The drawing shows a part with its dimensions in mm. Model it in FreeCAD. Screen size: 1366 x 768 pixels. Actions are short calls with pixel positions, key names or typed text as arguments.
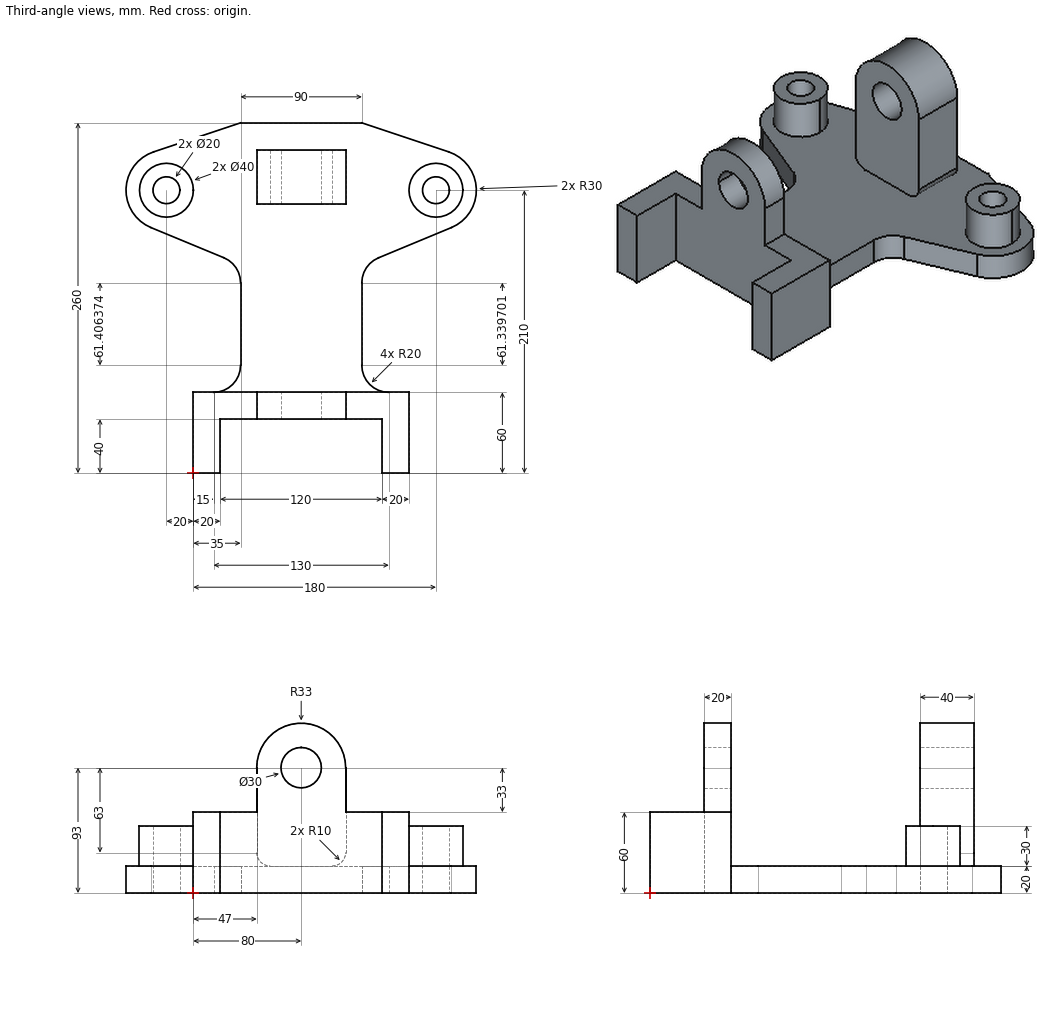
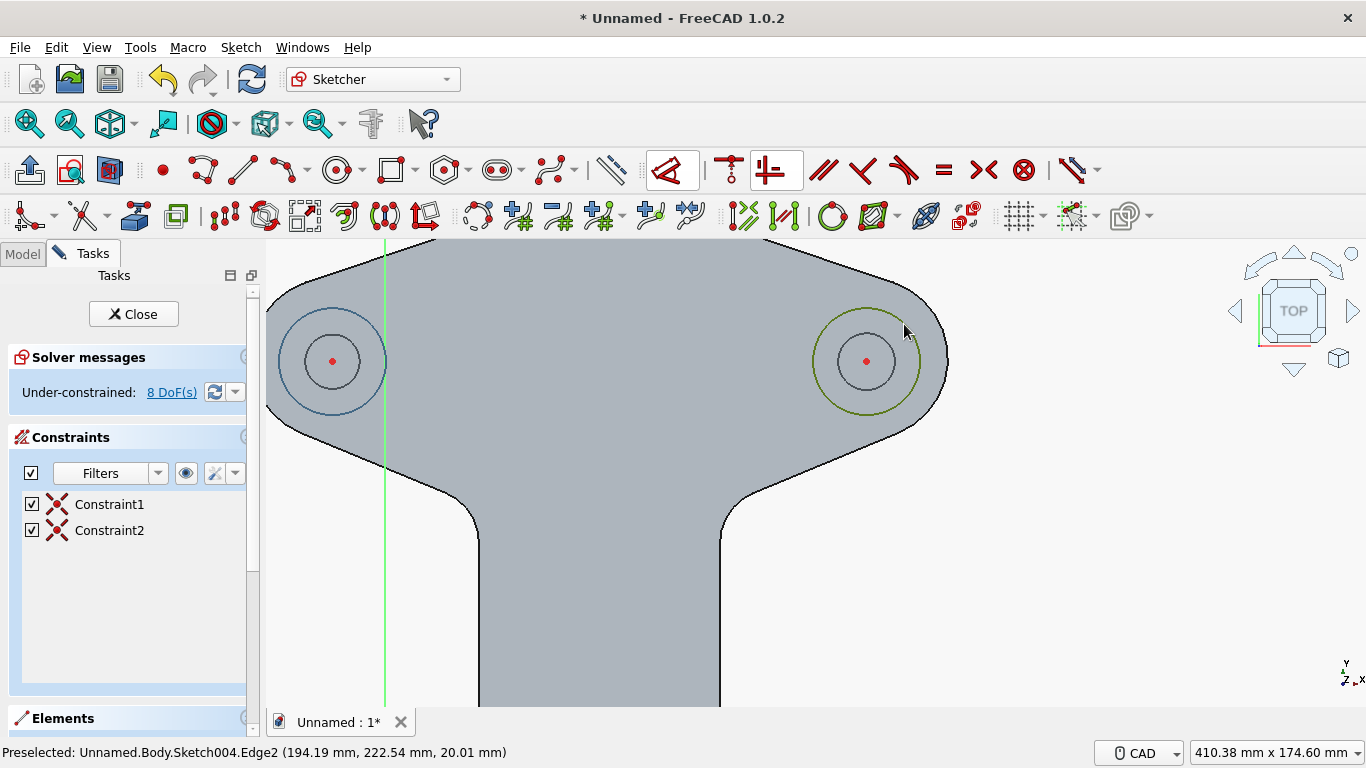
key(e)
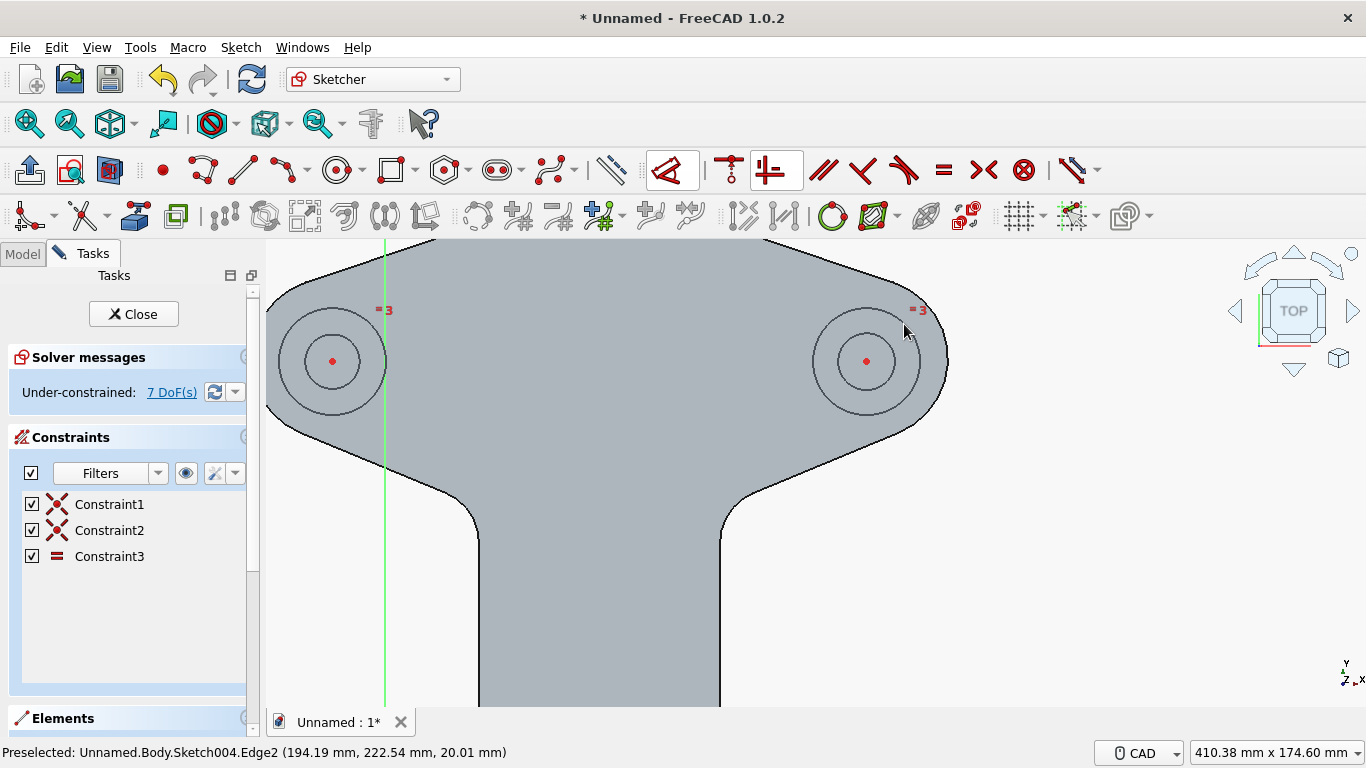
click(352, 342)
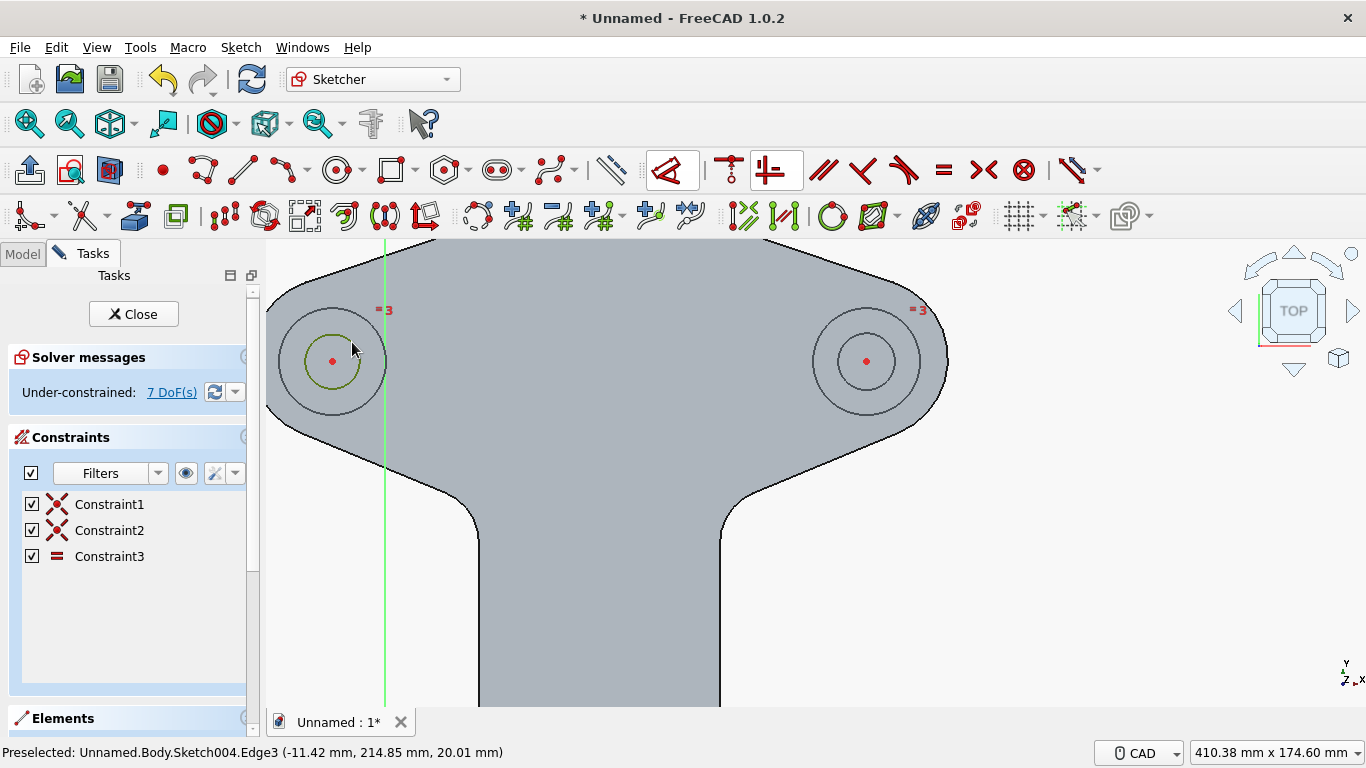
click(887, 342)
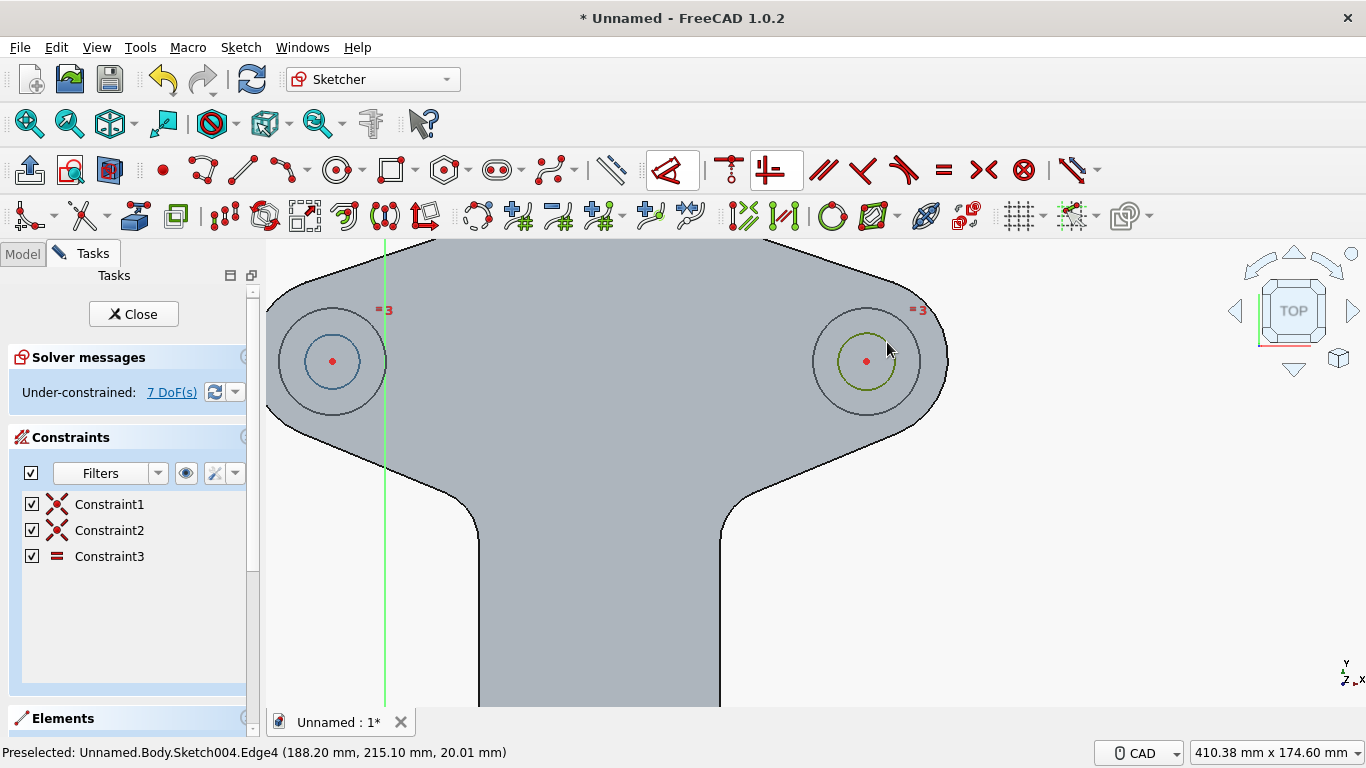
click(944, 170)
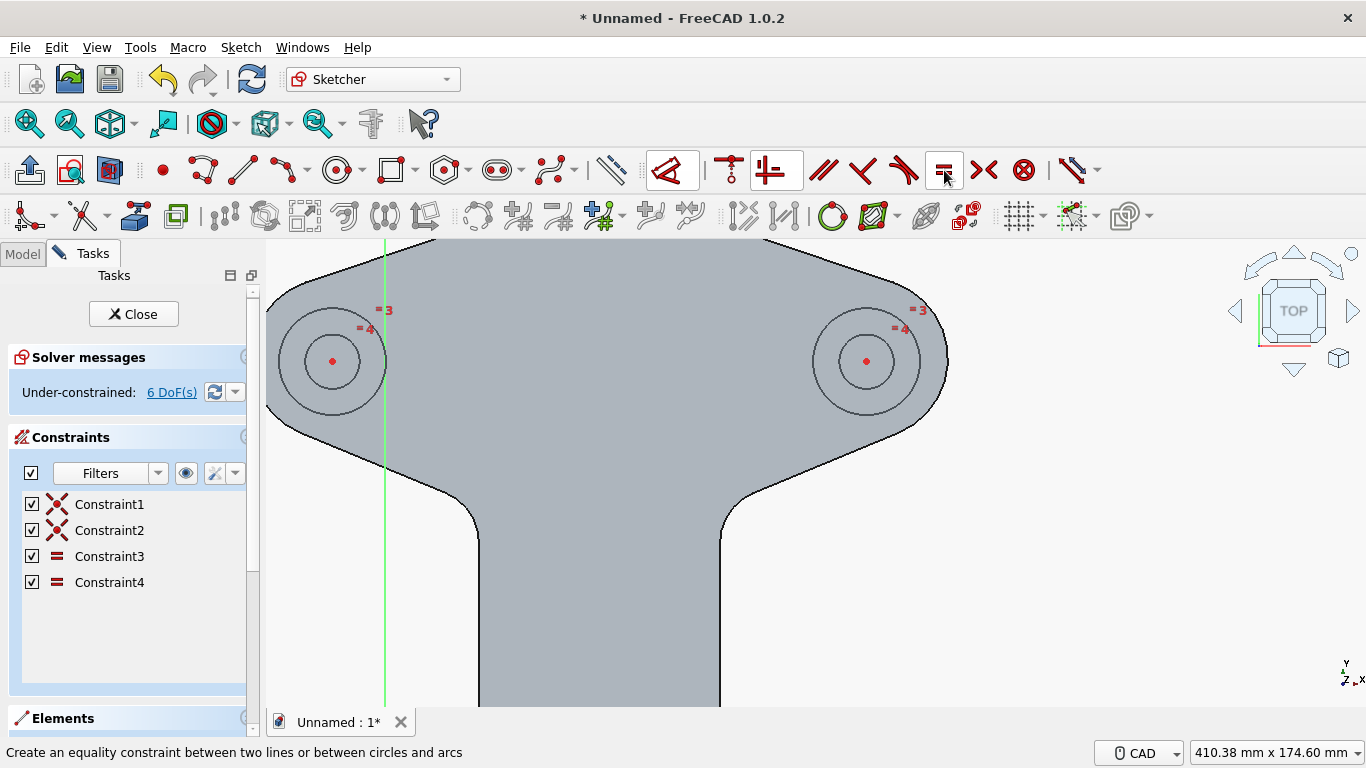
click(332, 362)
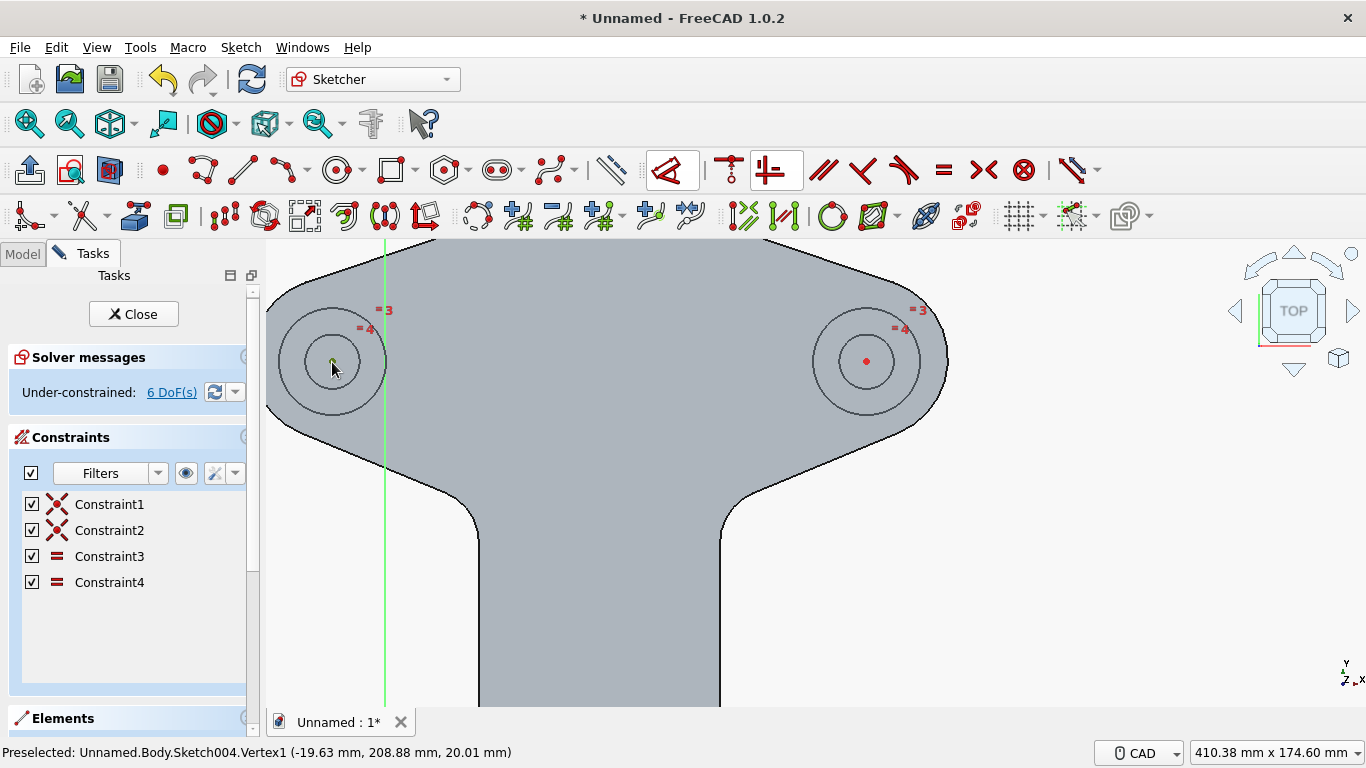
click(867, 362)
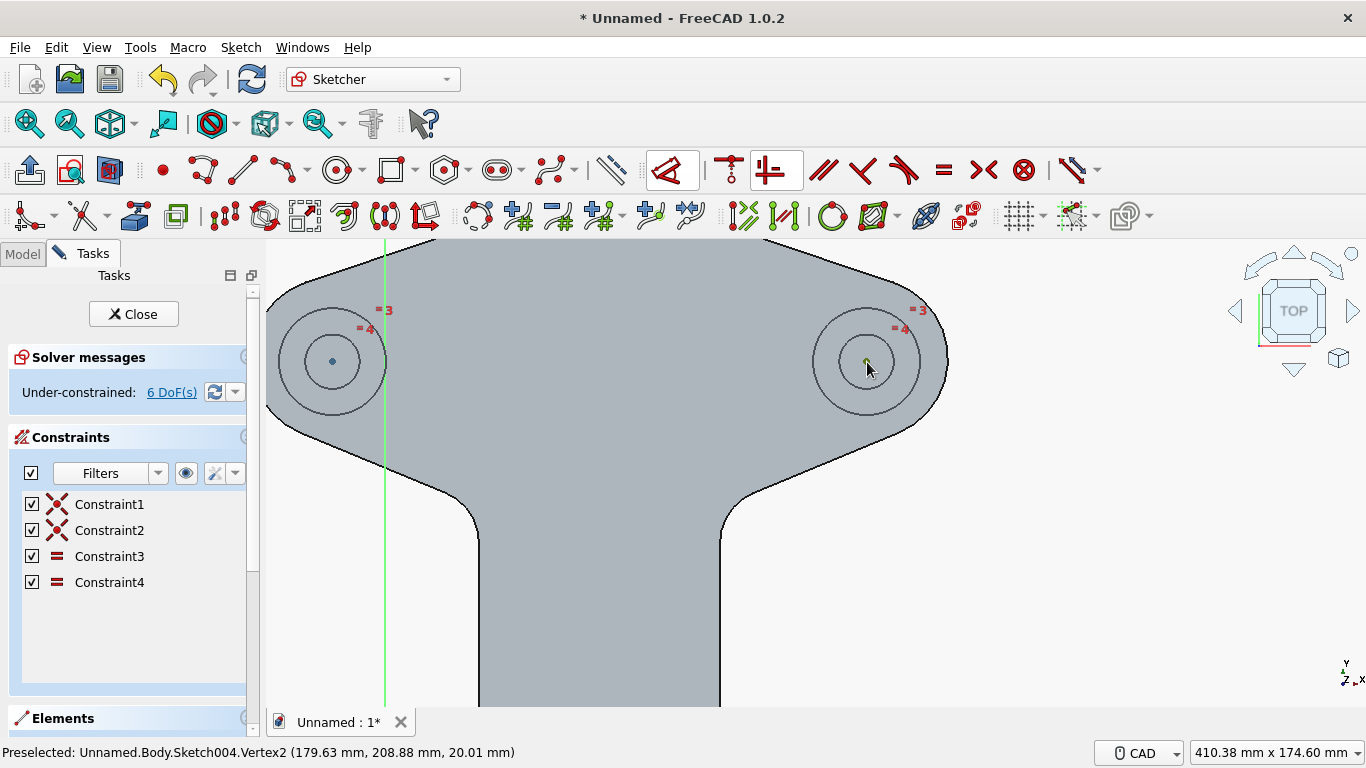
key(h)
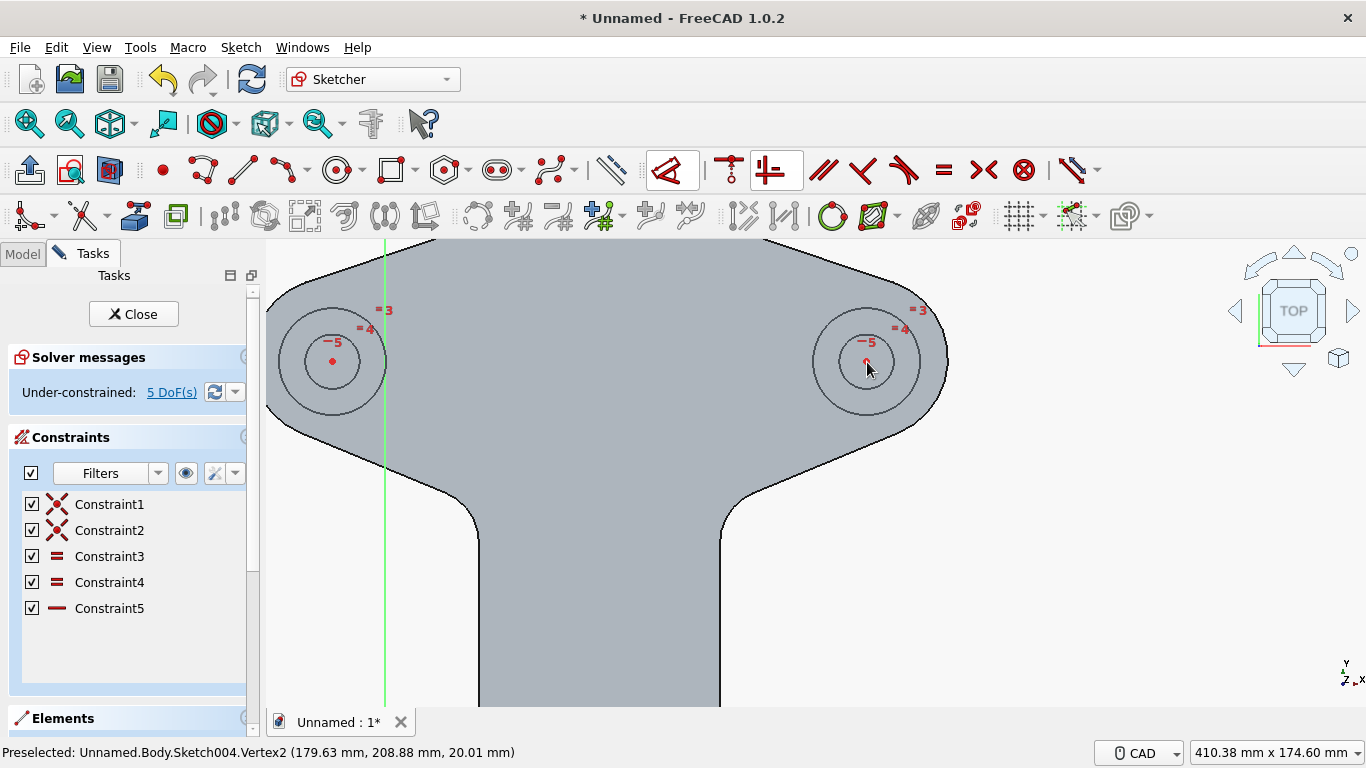
click(294, 324)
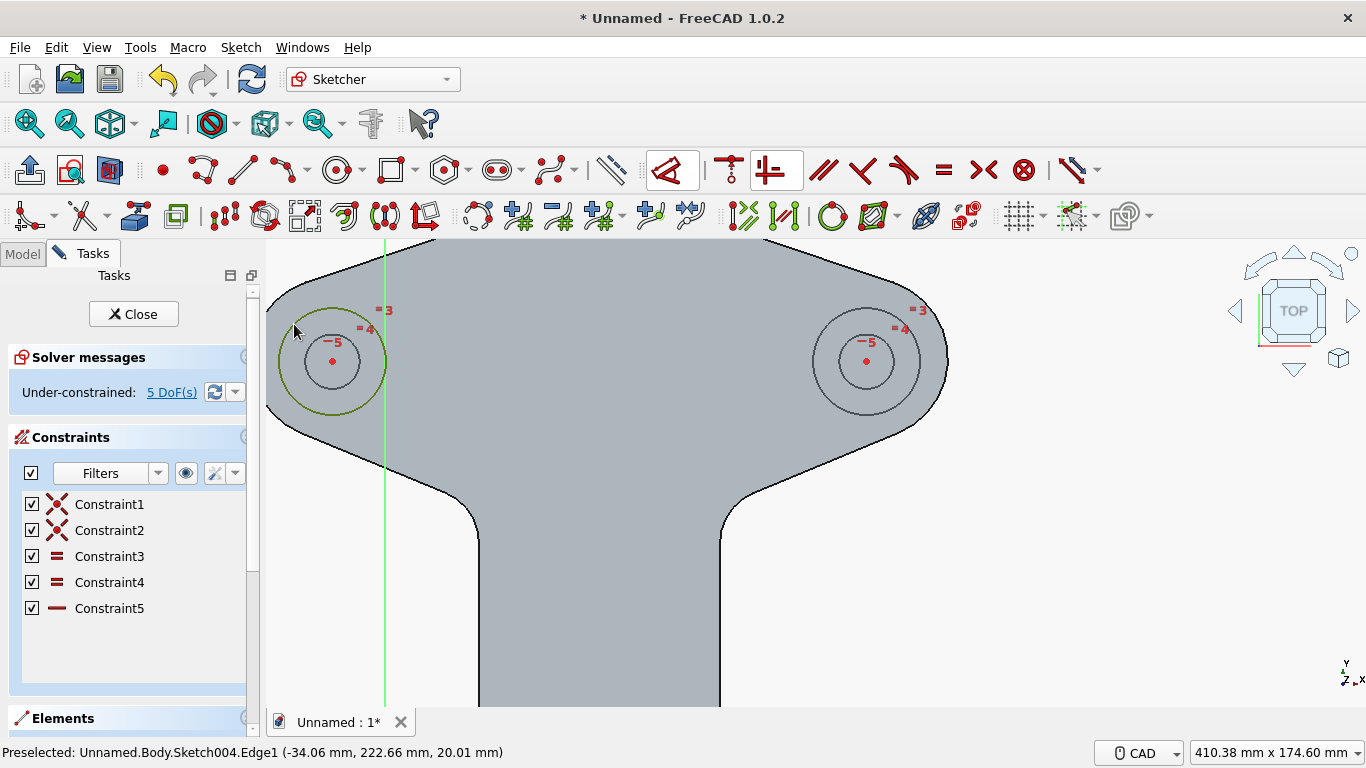
key(k)
key(o)